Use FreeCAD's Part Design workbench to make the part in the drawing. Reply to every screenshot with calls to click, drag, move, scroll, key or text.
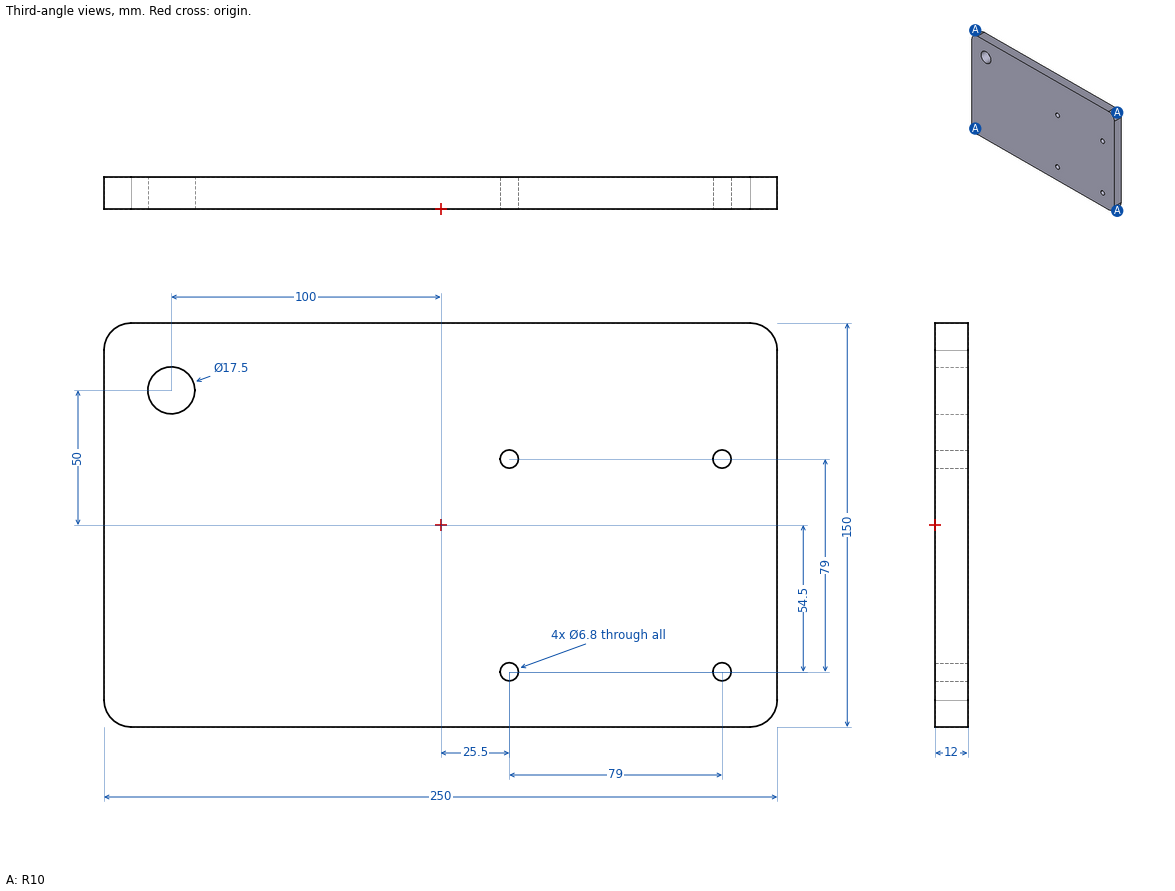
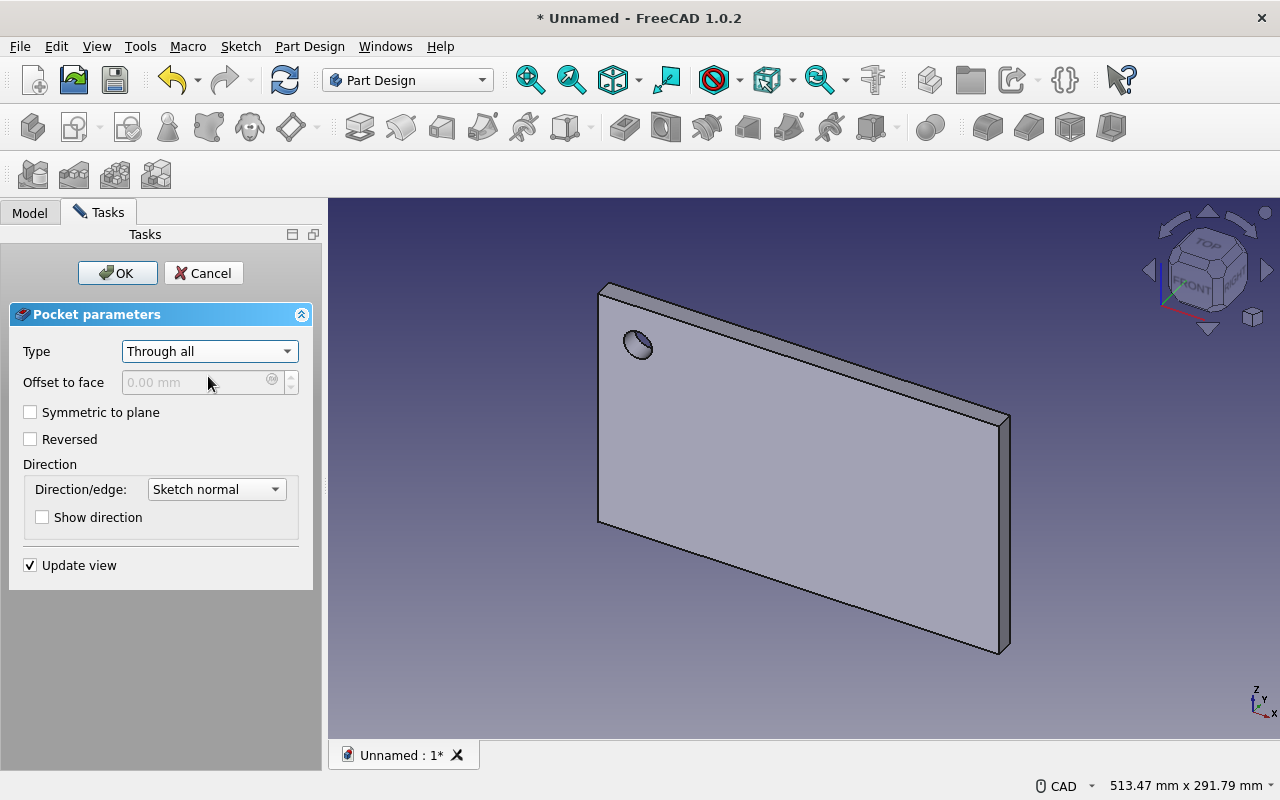
click(118, 273)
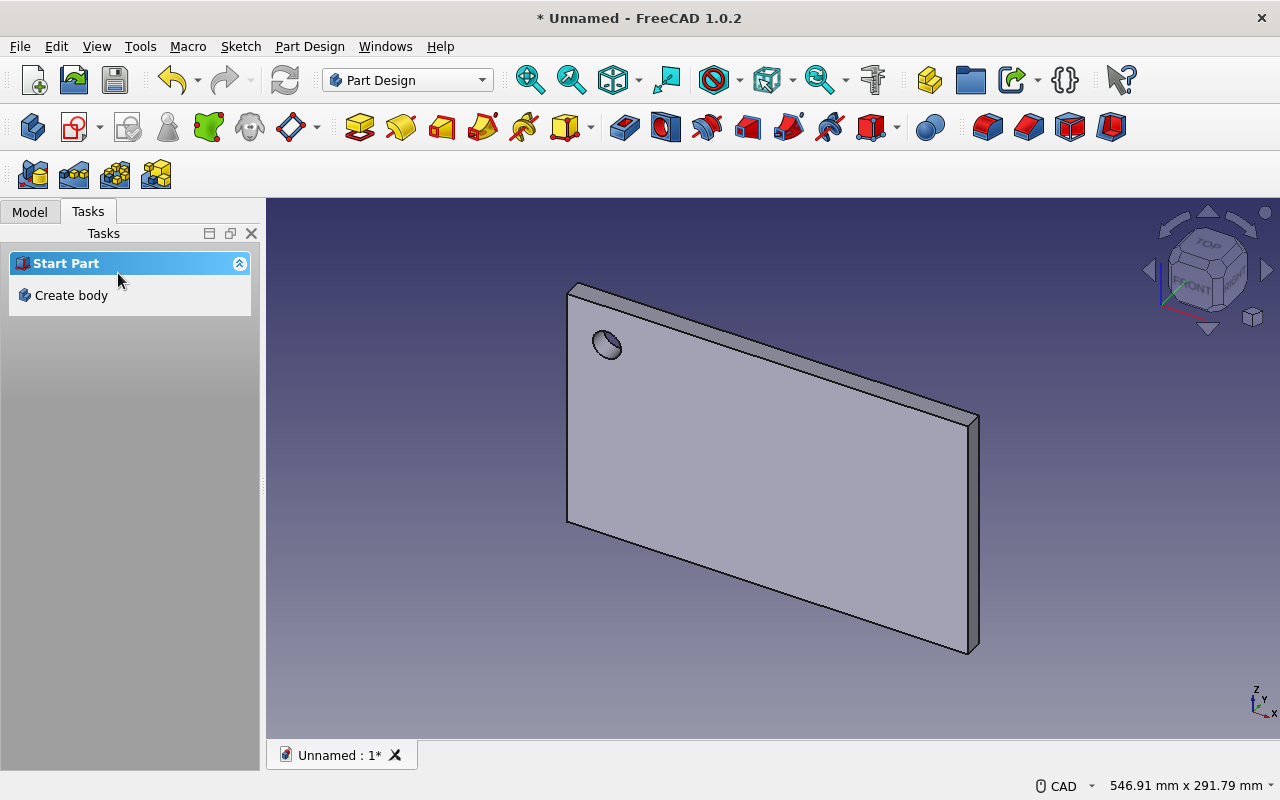
key(4)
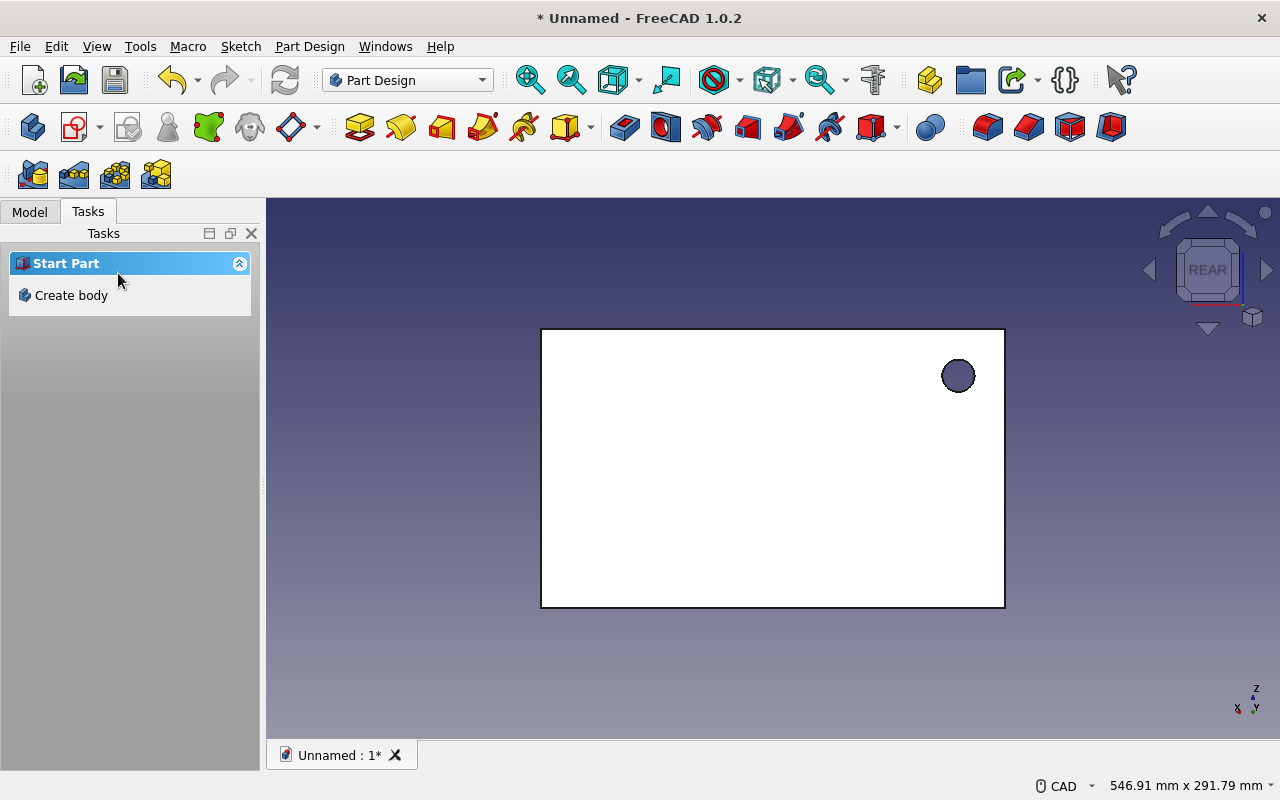
click(707, 467)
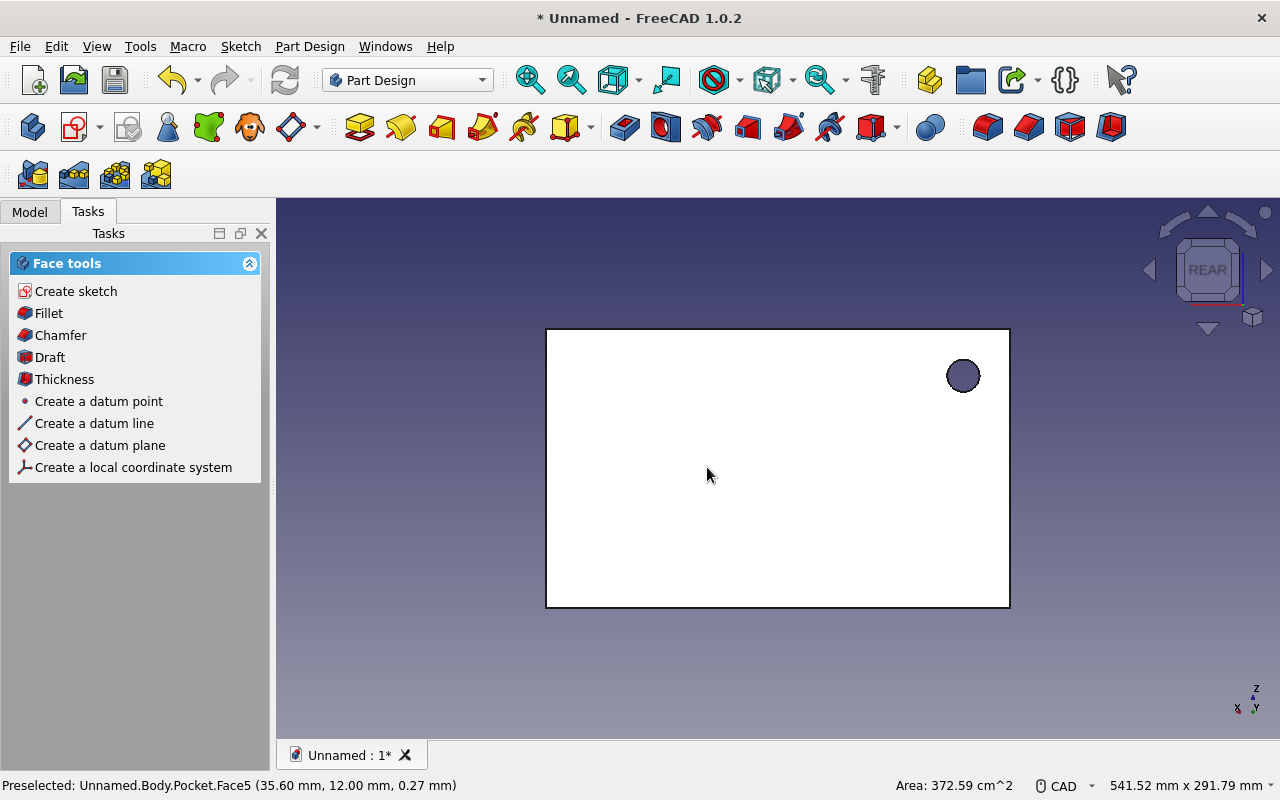
click(74, 128)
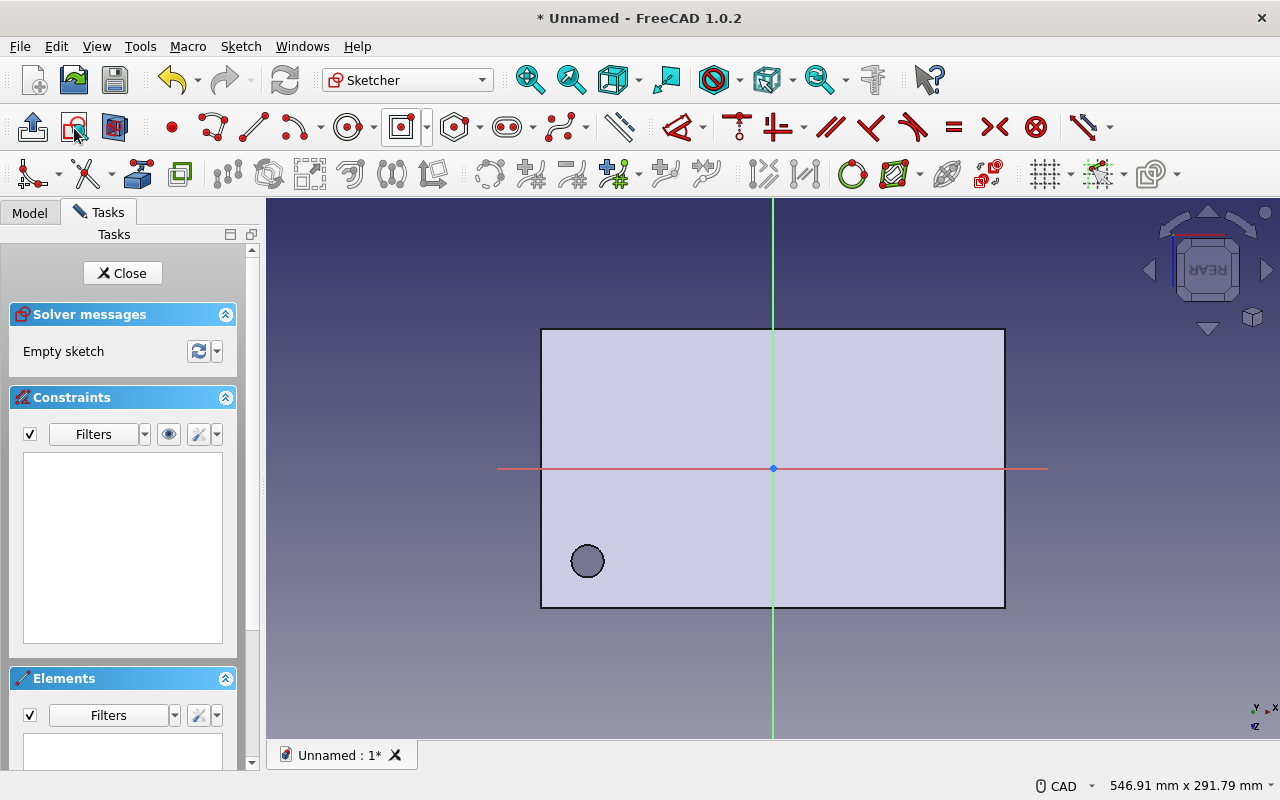
scroll(1011, 418, up, 4)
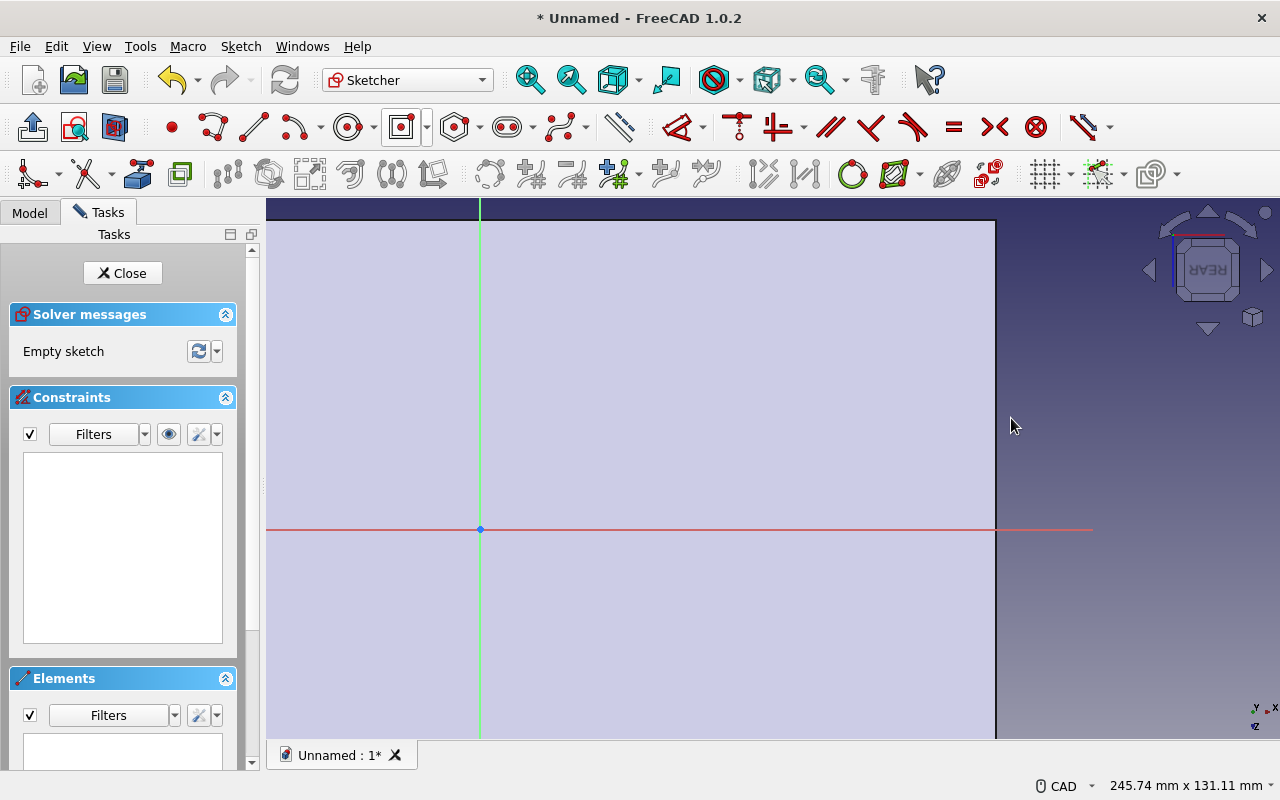
click(348, 128)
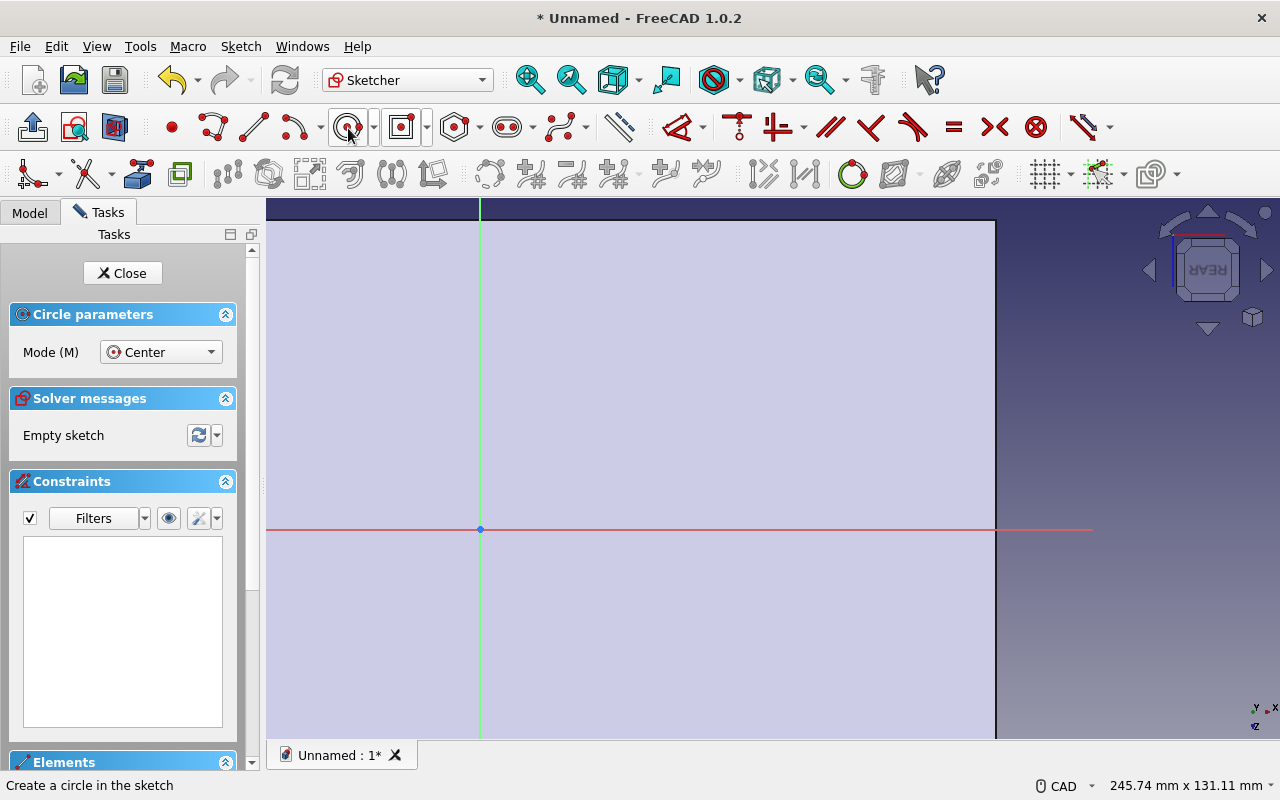
scroll(586, 305, up, 3)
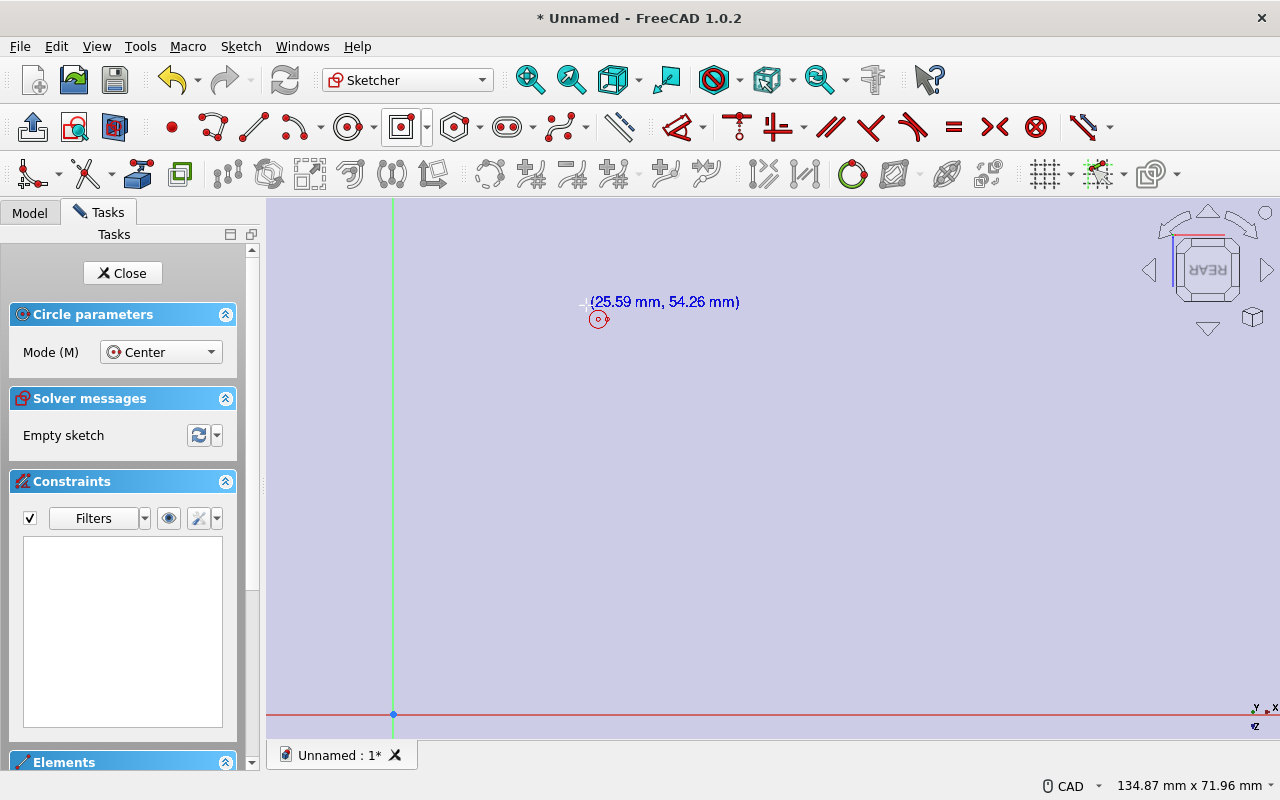
click(585, 305)
move(603, 287)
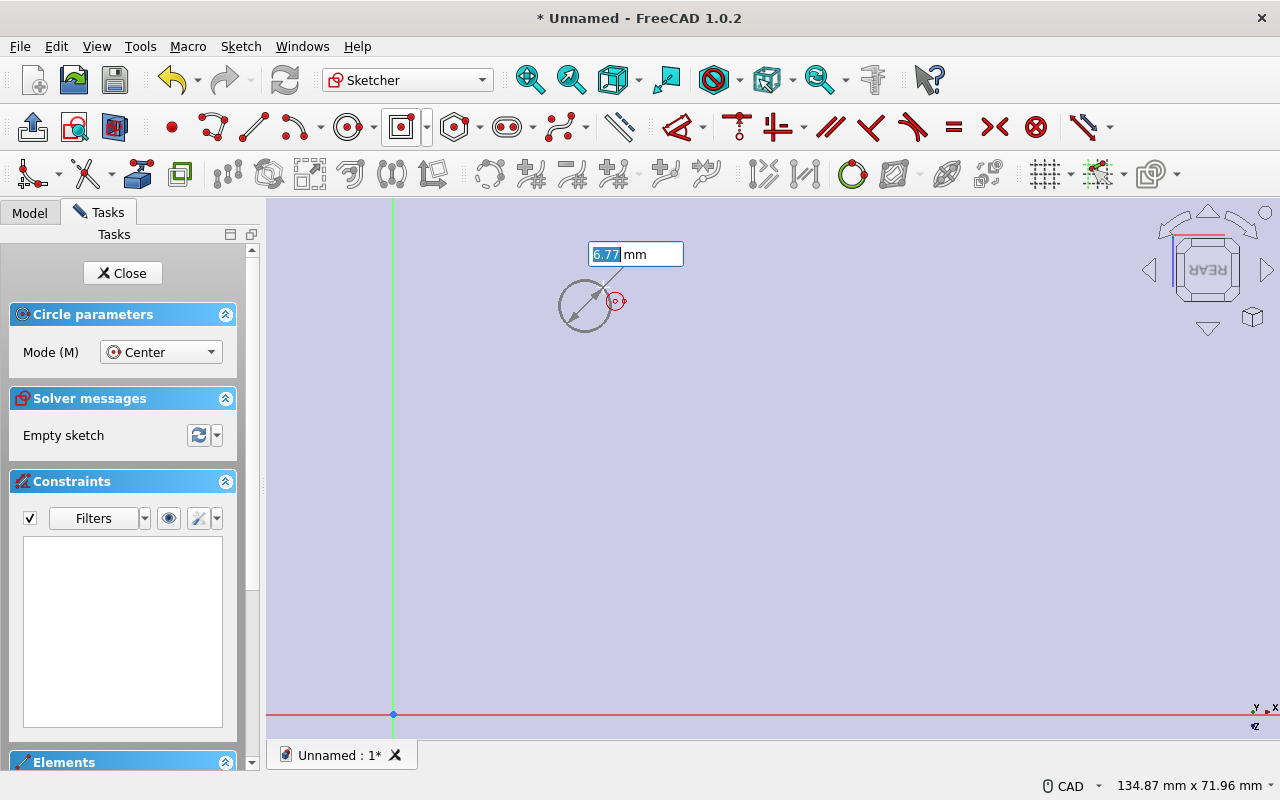
text(6.8)
key(Return)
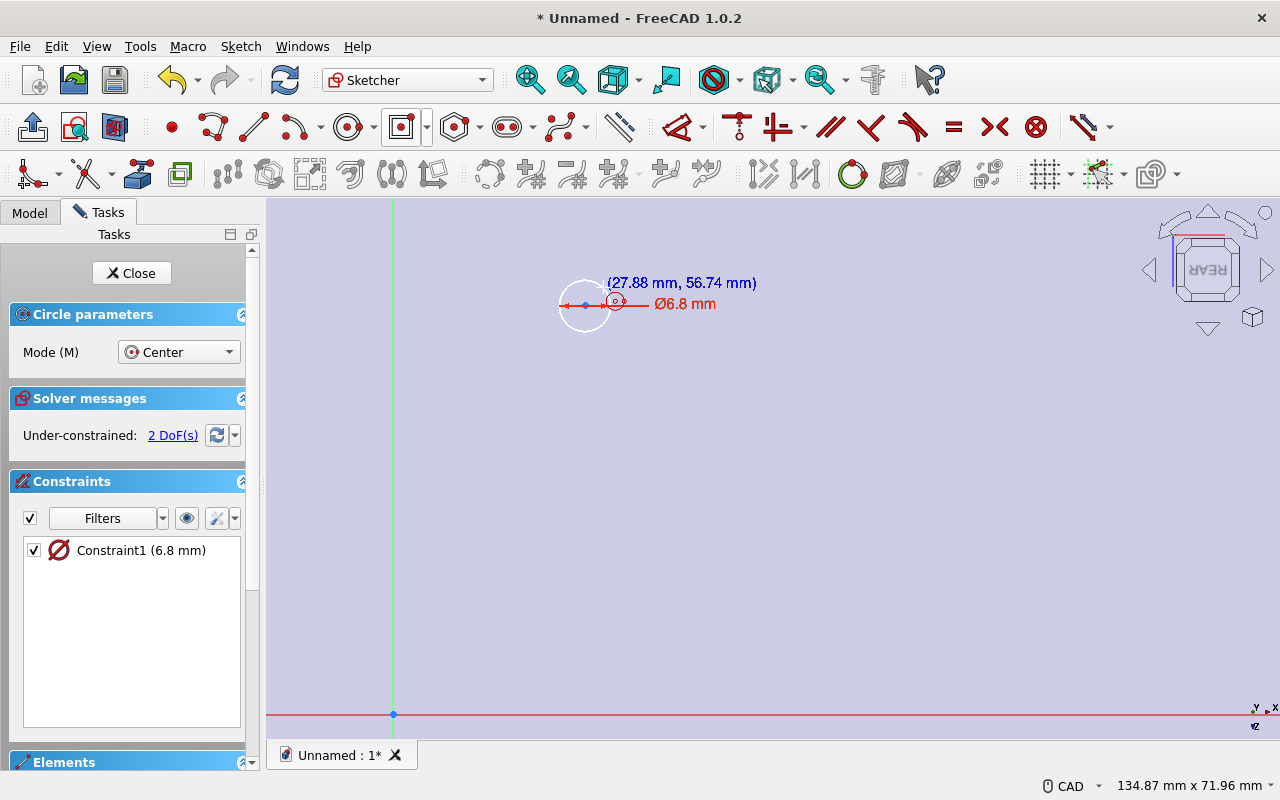
scroll(590, 306, down, 3)